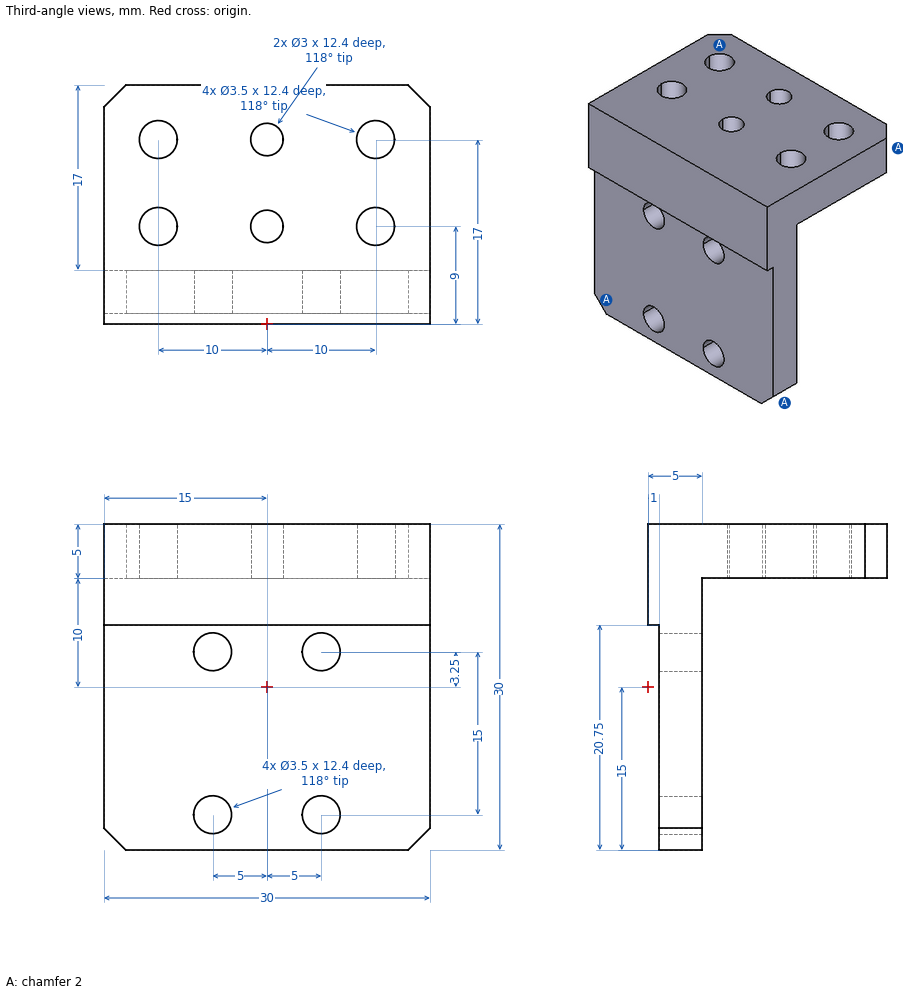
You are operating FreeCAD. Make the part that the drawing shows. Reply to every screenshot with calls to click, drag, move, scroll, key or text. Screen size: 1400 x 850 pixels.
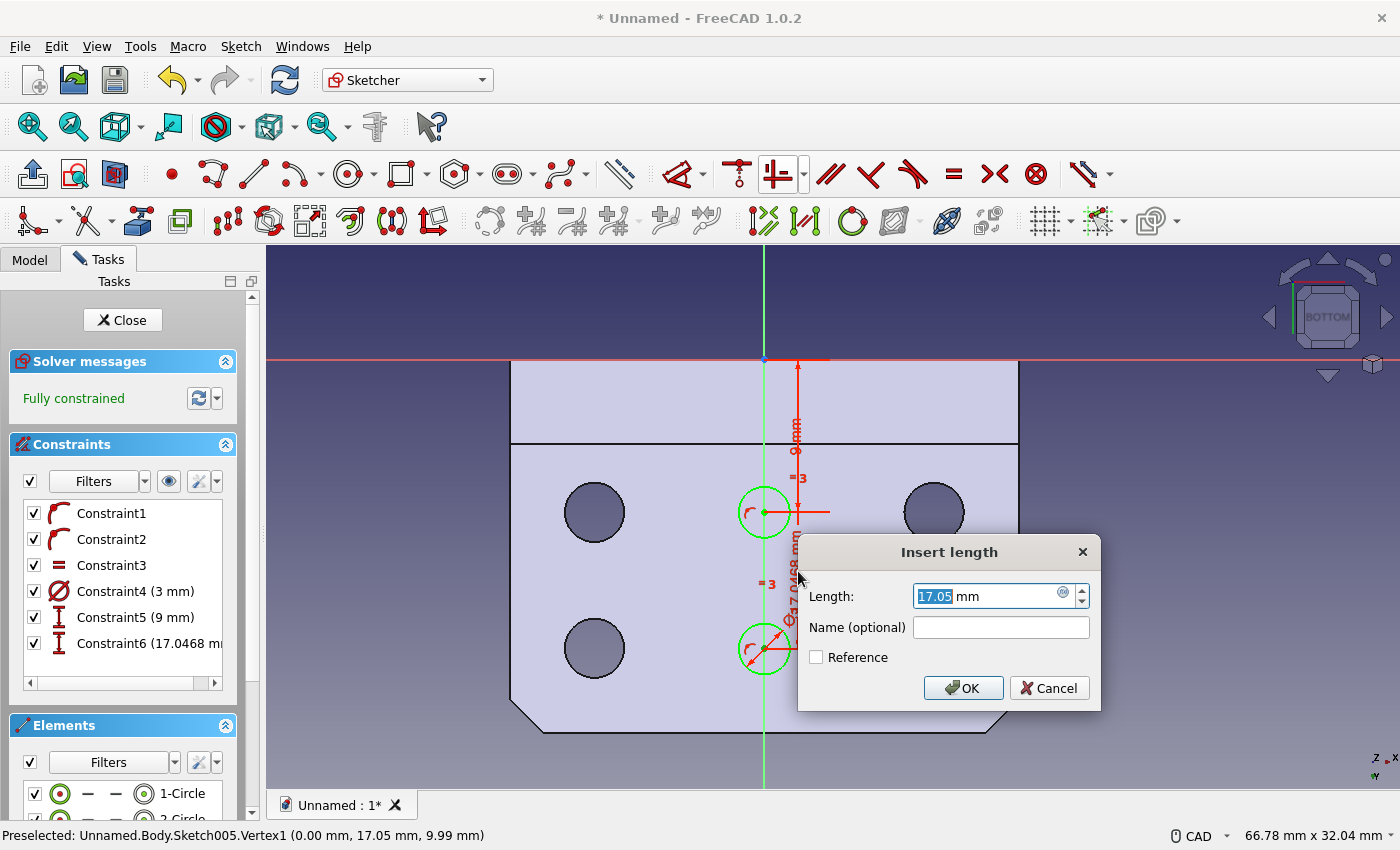
text(17)
key(Return)
key(Escape)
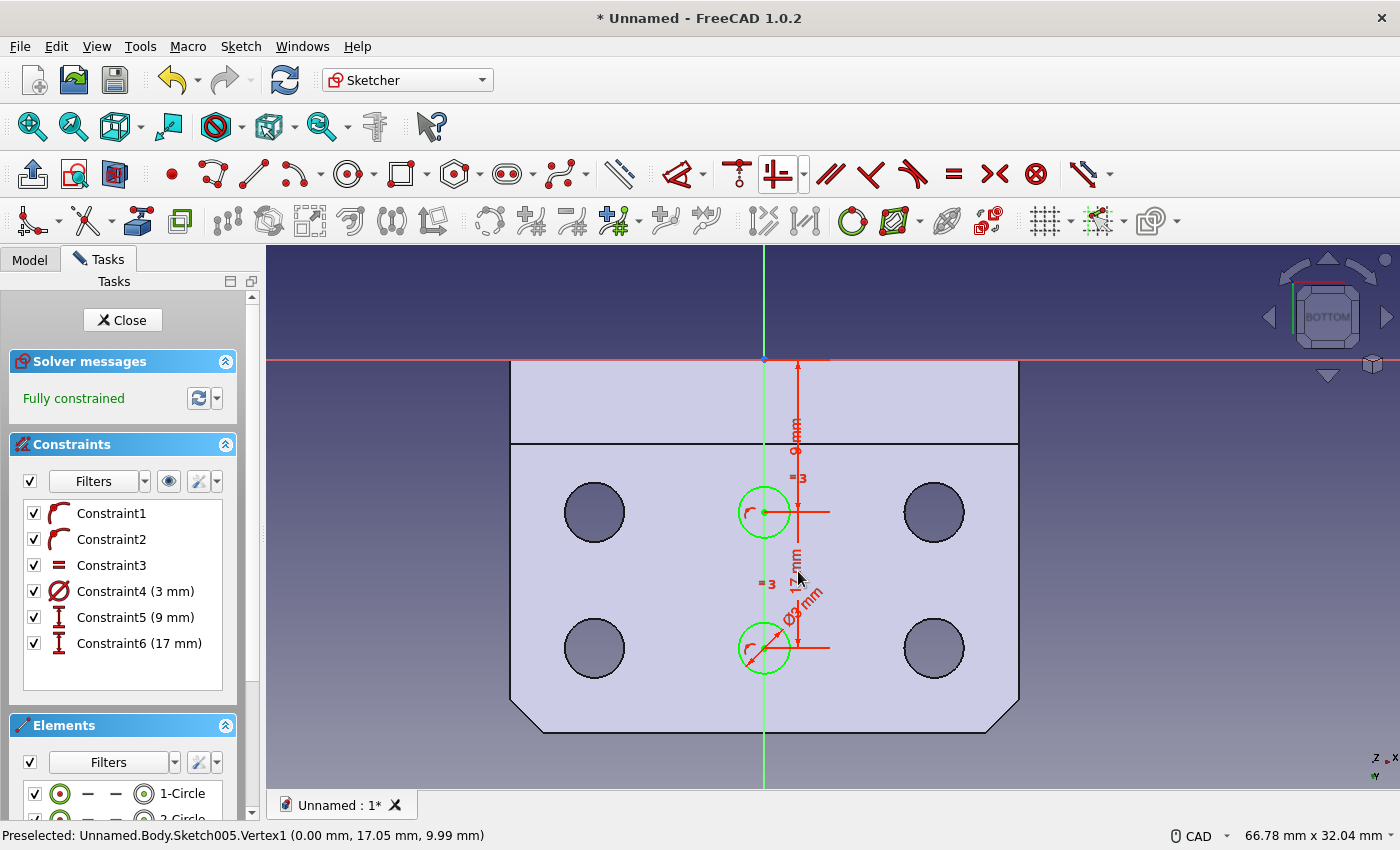
click(123, 320)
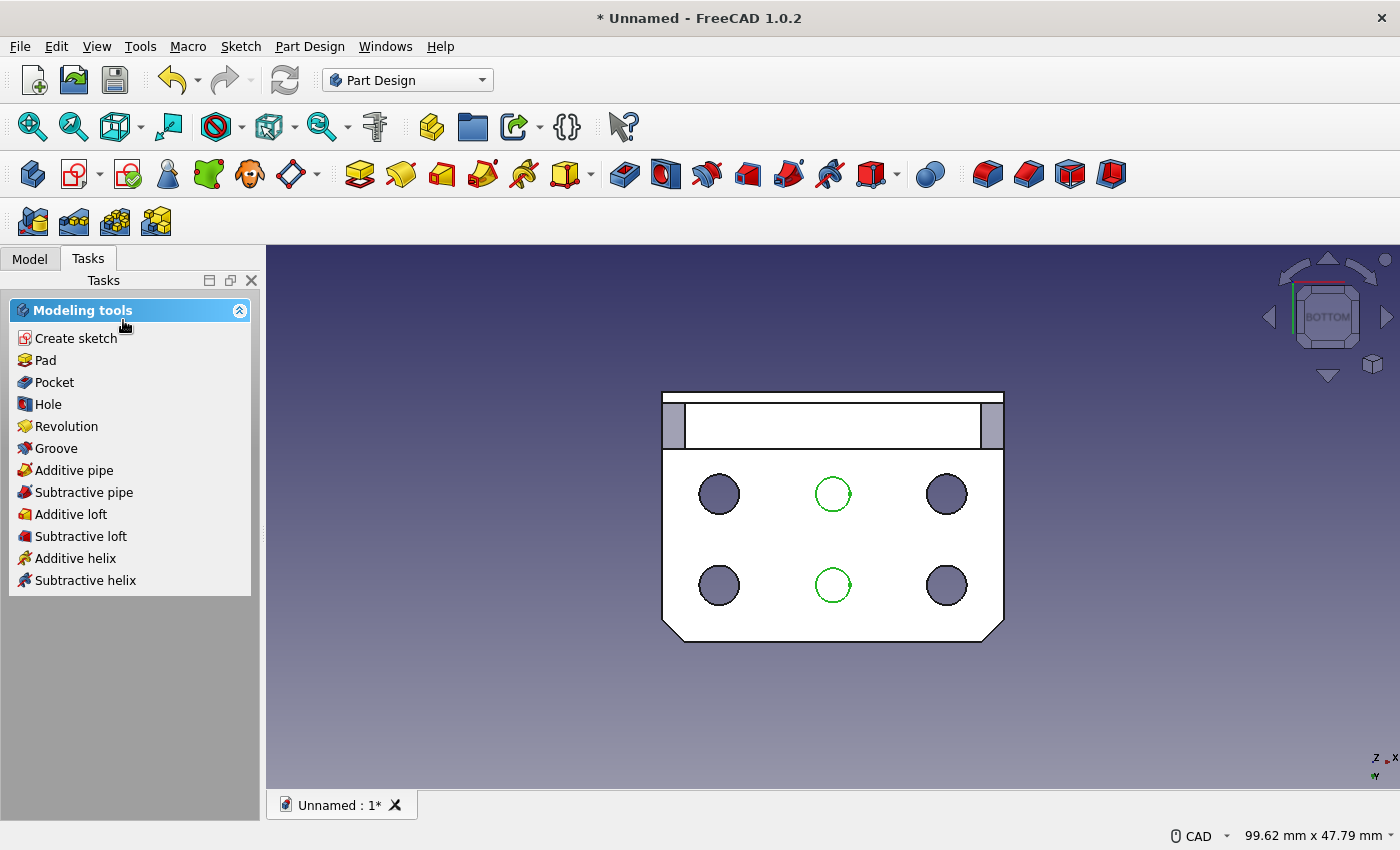
click(666, 174)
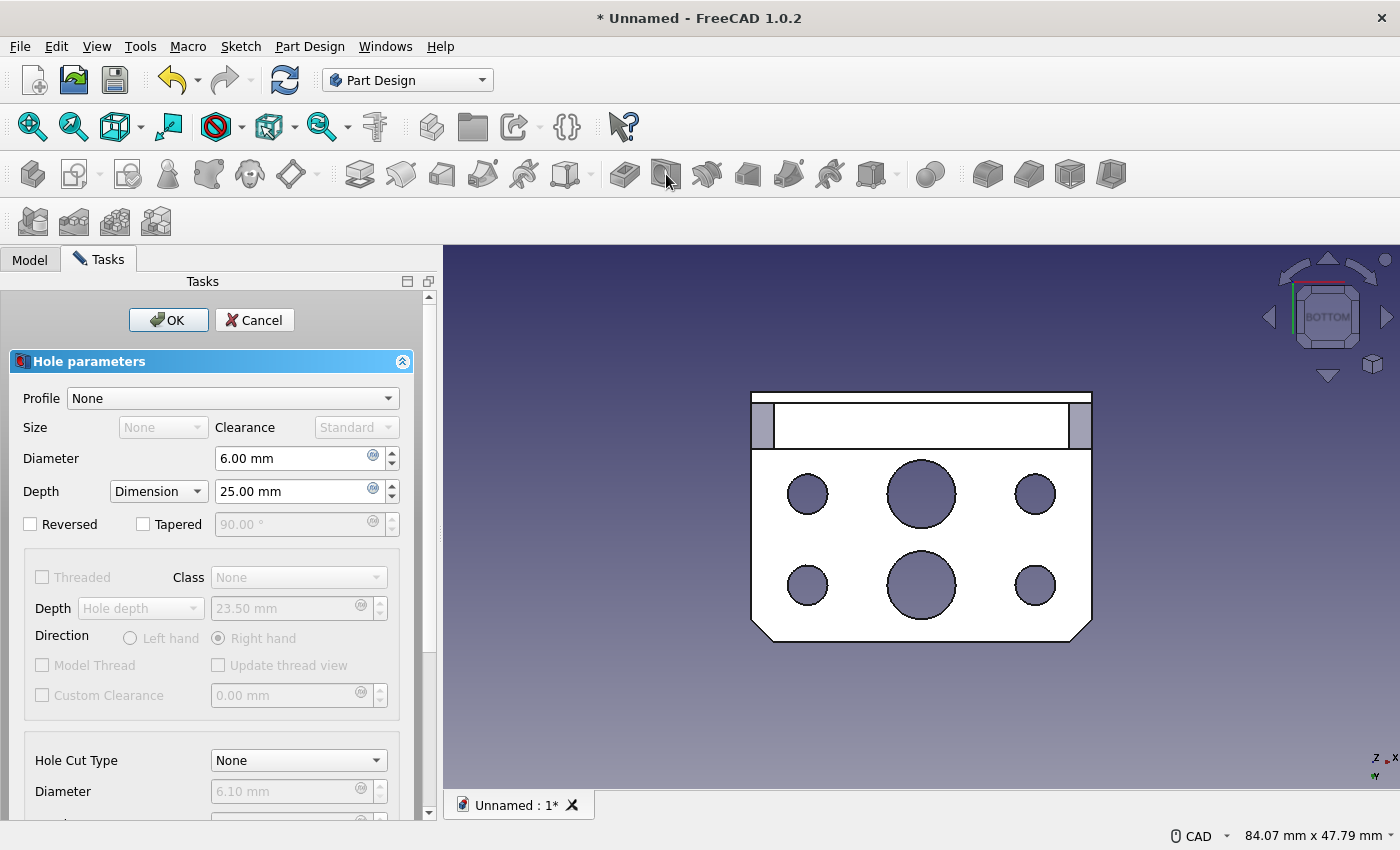
triple_click(300, 458)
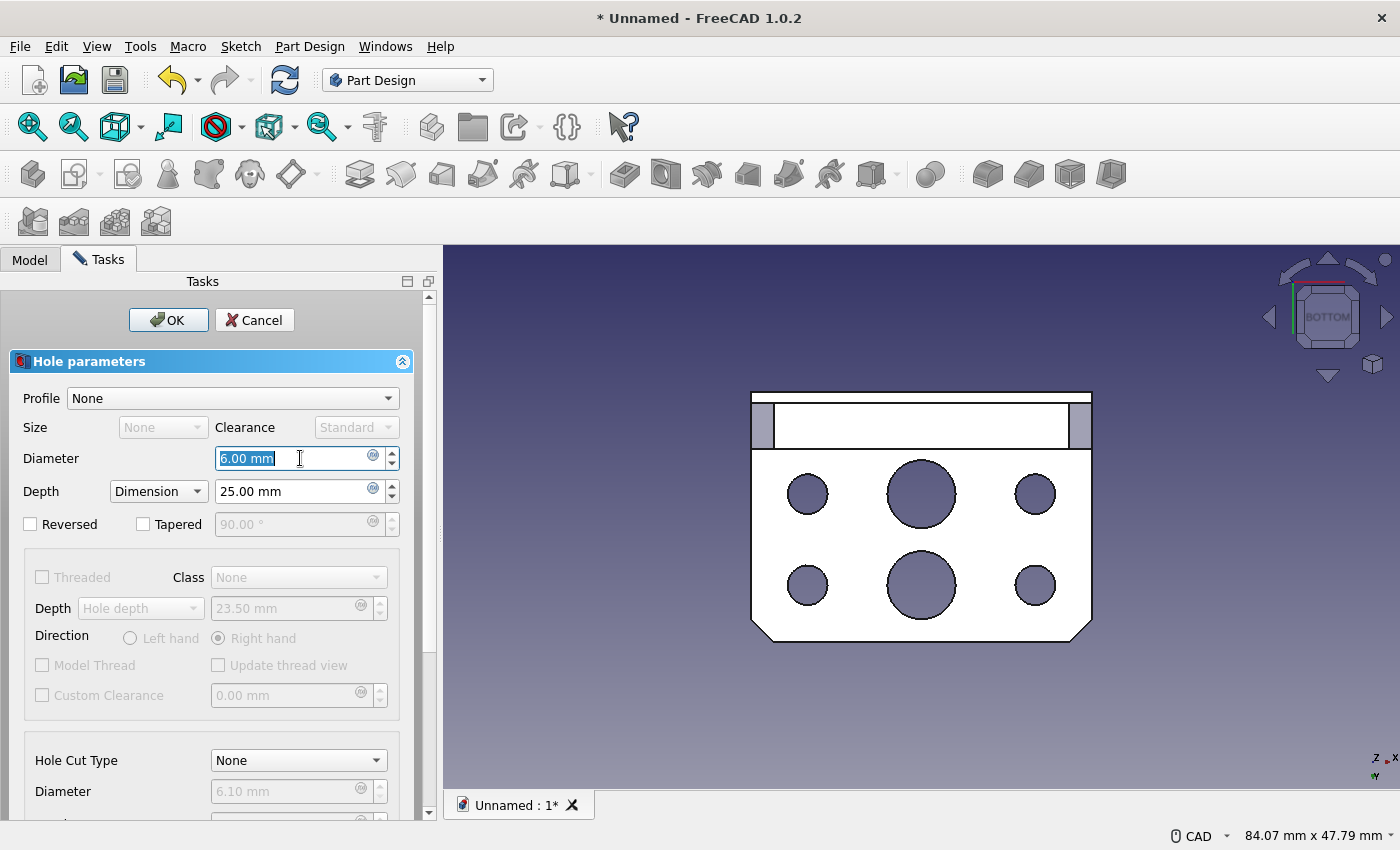
text(3)
key(Tab)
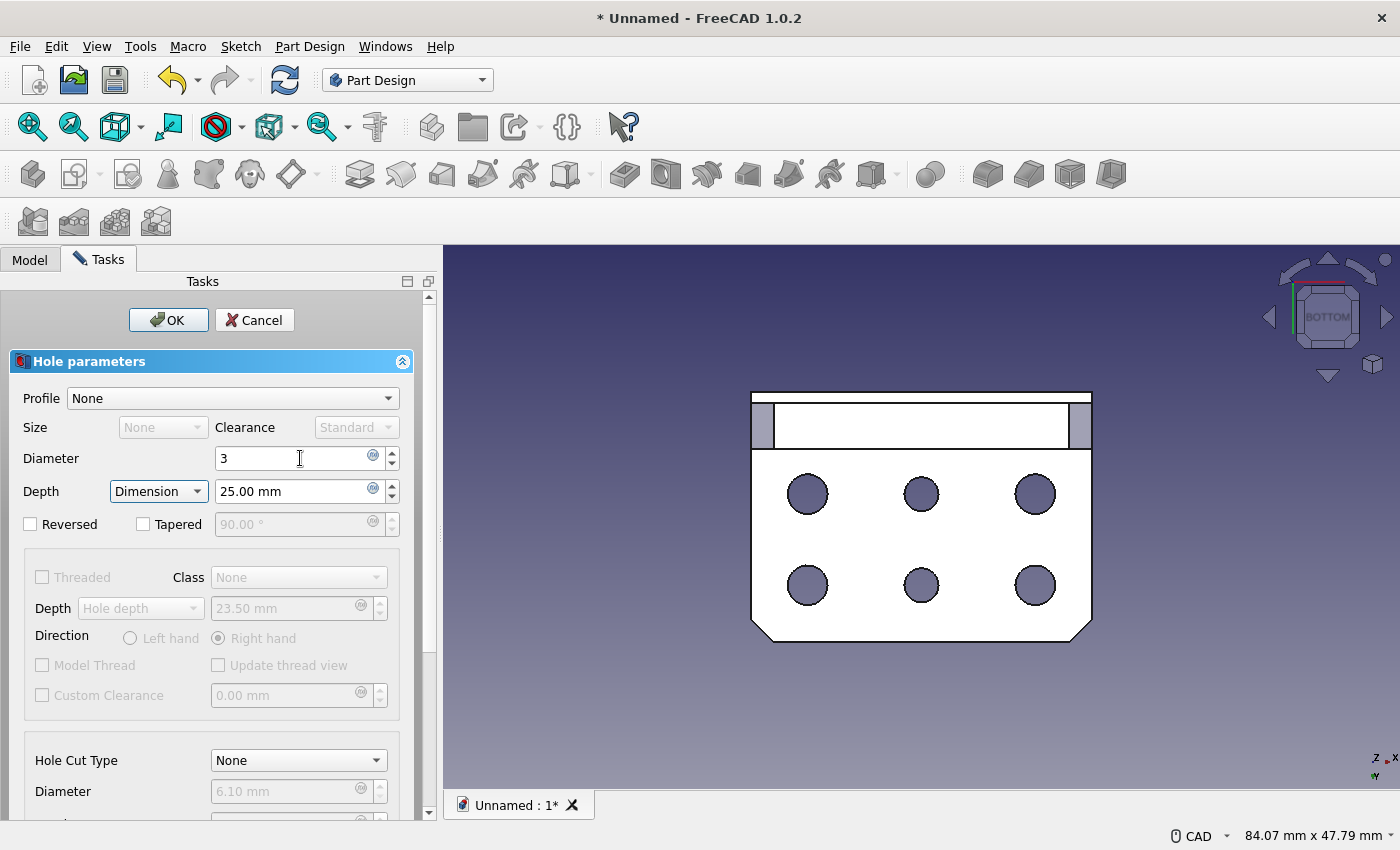
triple_click(300, 492)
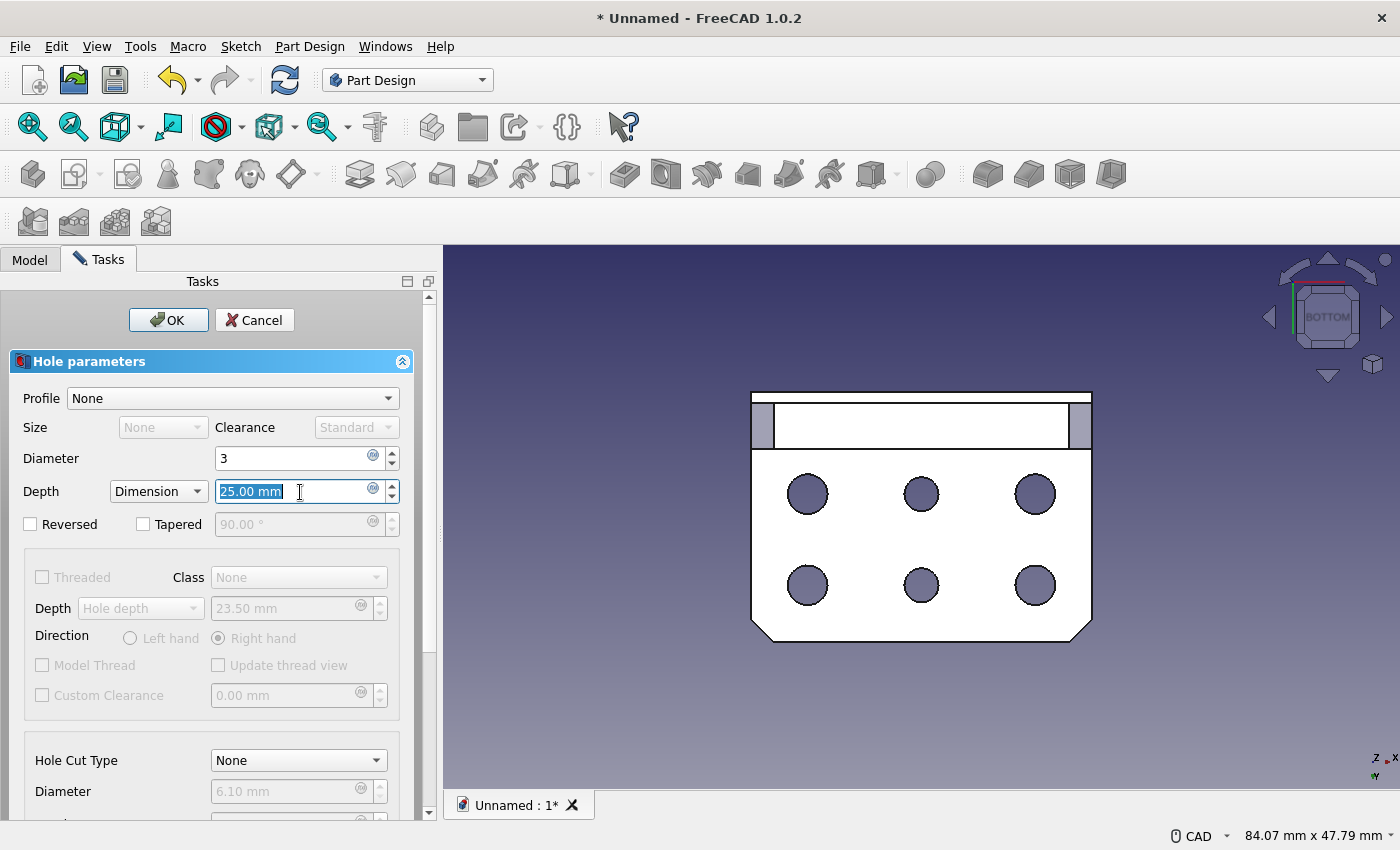
text(12.4)
key(Tab)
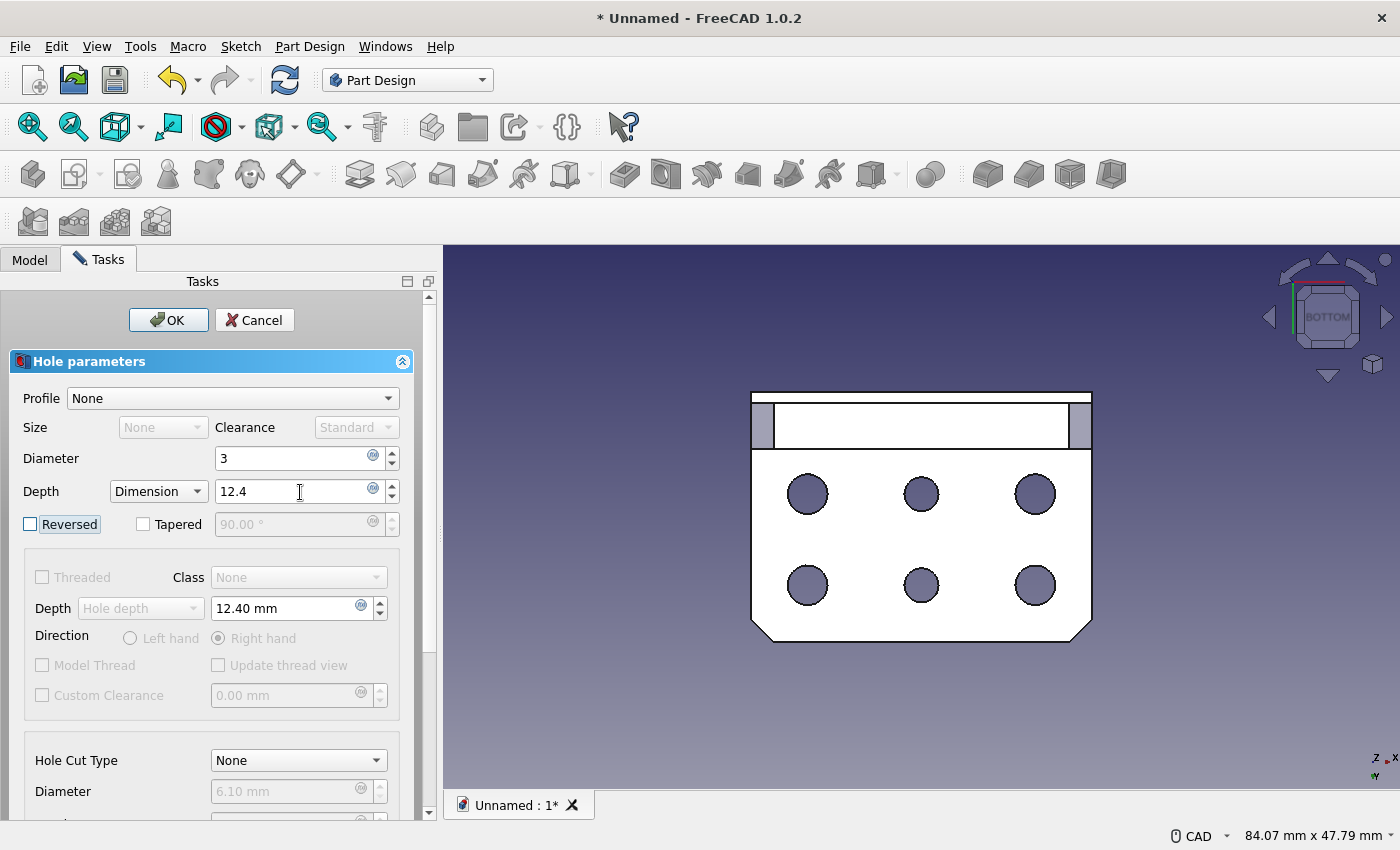
click(169, 320)